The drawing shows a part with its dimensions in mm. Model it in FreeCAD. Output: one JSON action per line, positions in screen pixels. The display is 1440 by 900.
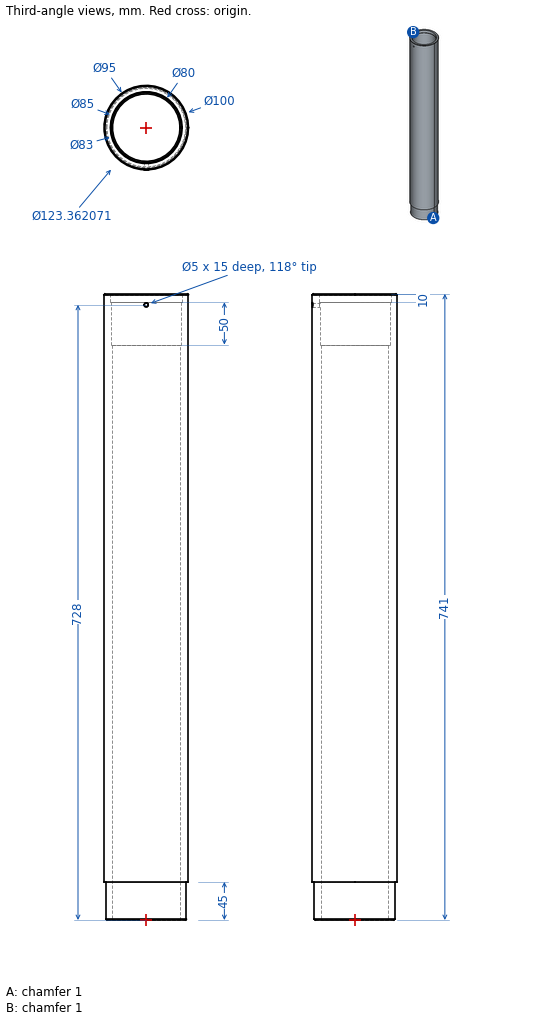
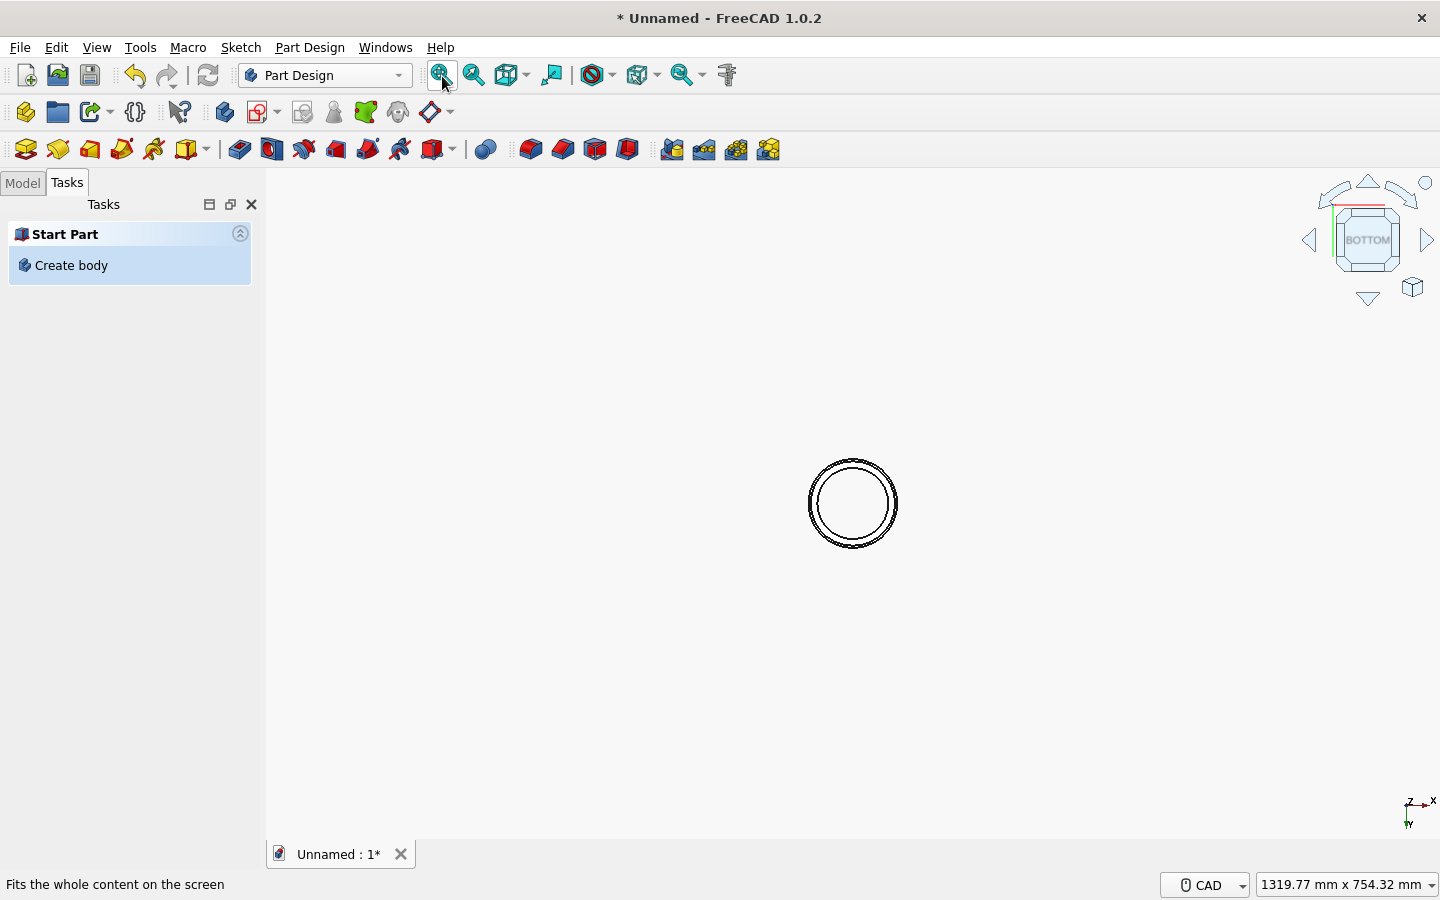
{"action": "left_click", "coordinate": [811, 502]}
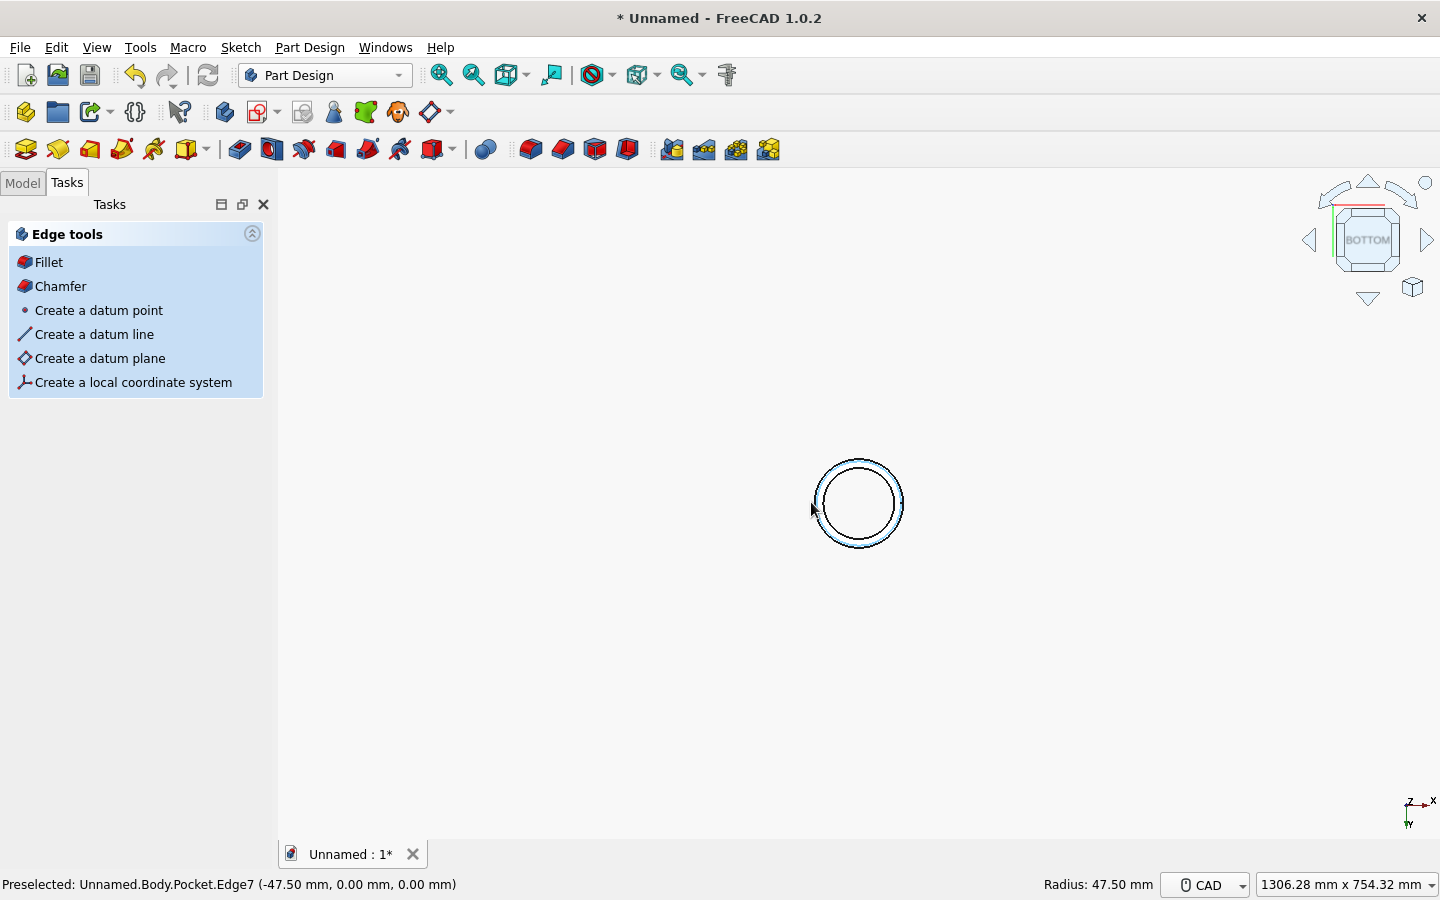
{"action": "left_click", "coordinate": [564, 150]}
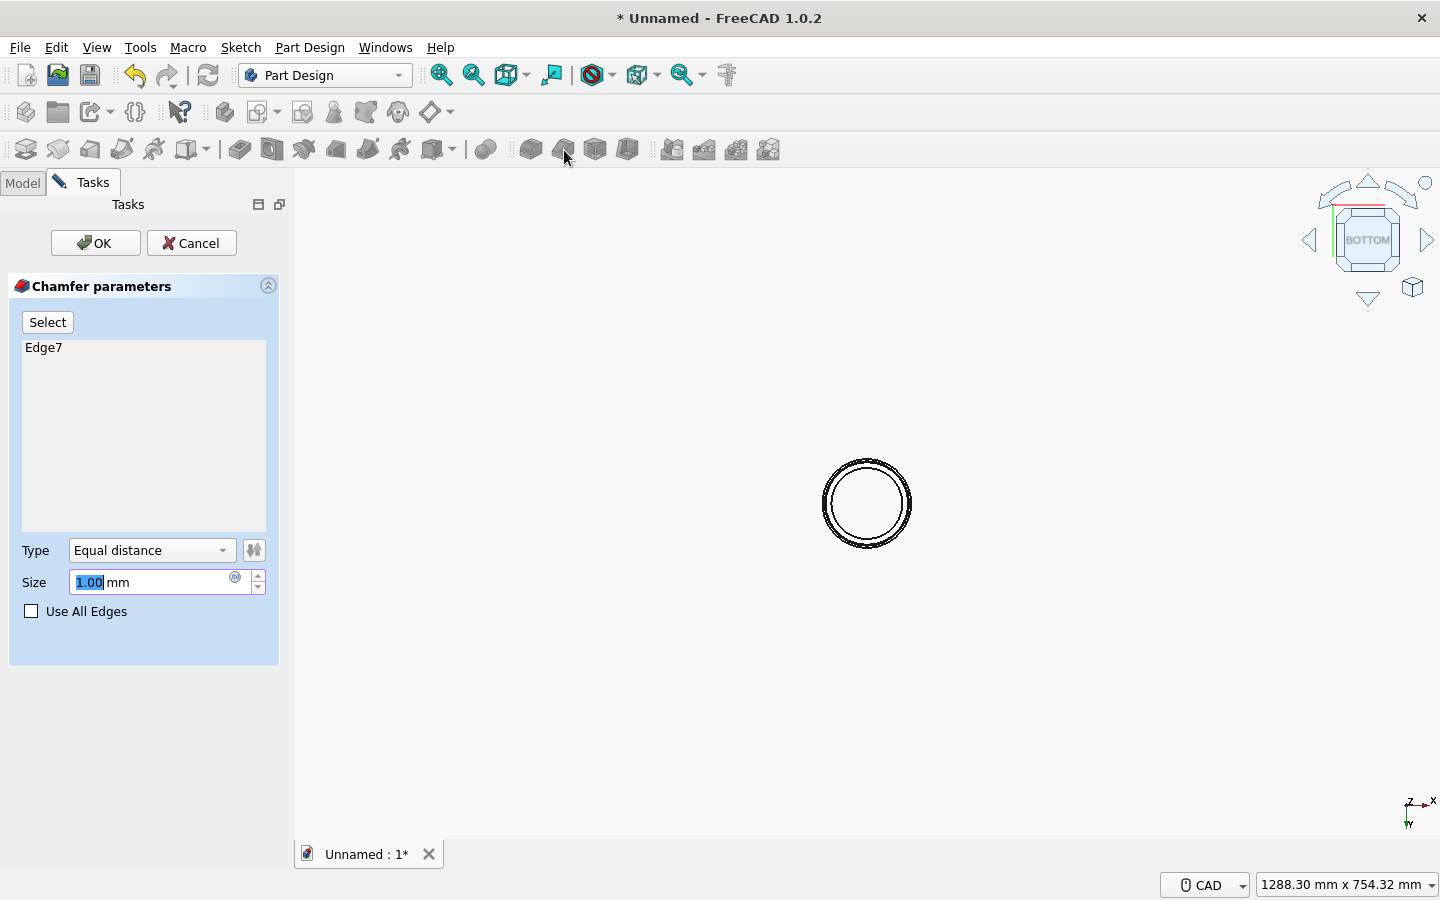
{"action": "type", "text": "1"}
{"action": "key", "text": "Tab"}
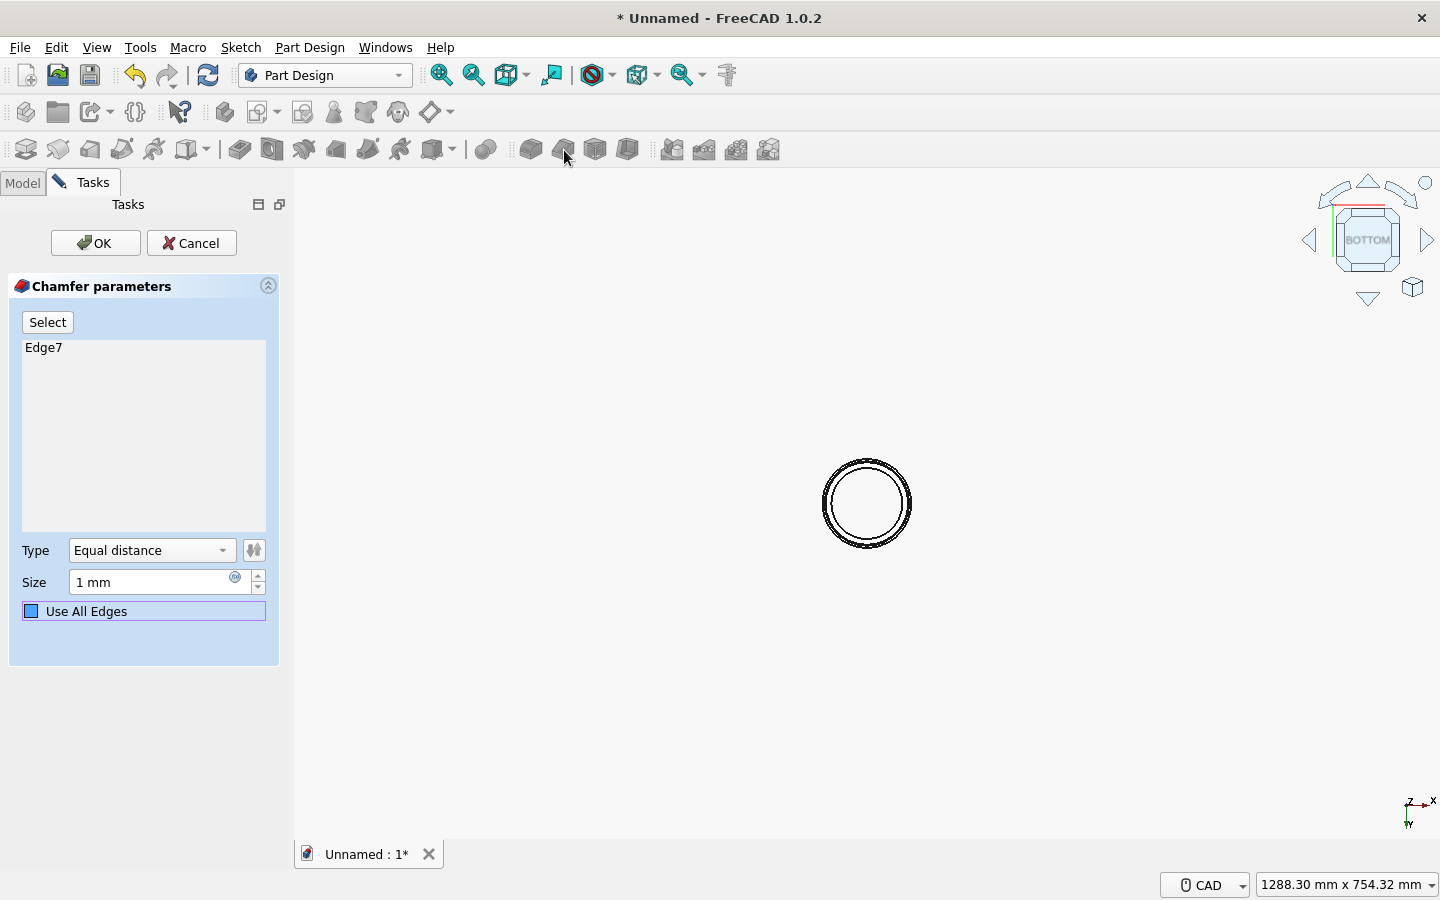
{"action": "left_click", "coordinate": [96, 243]}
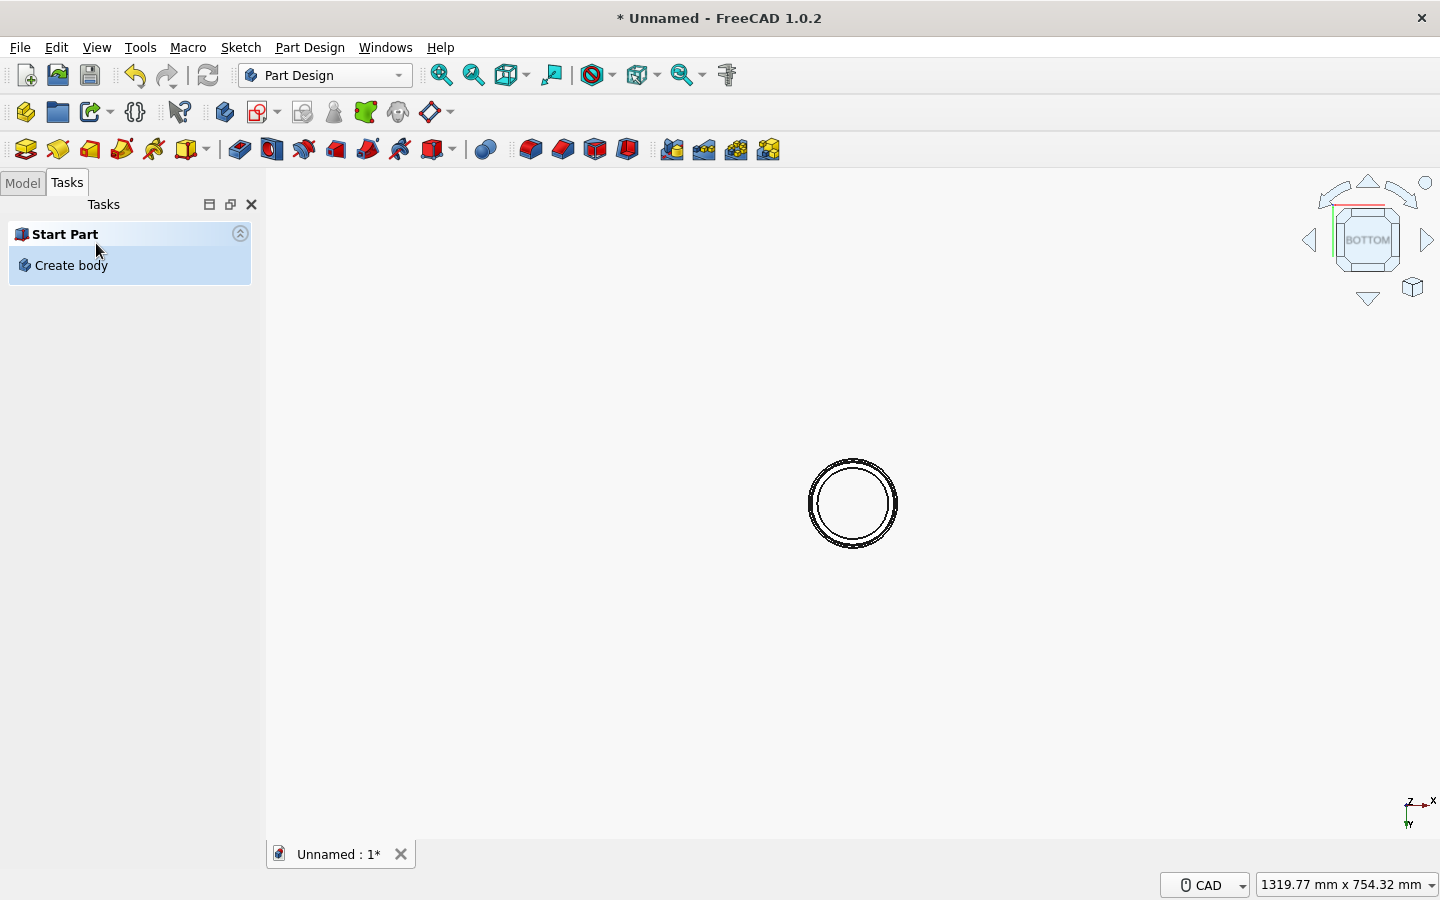
{"action": "left_click", "coordinate": [442, 76]}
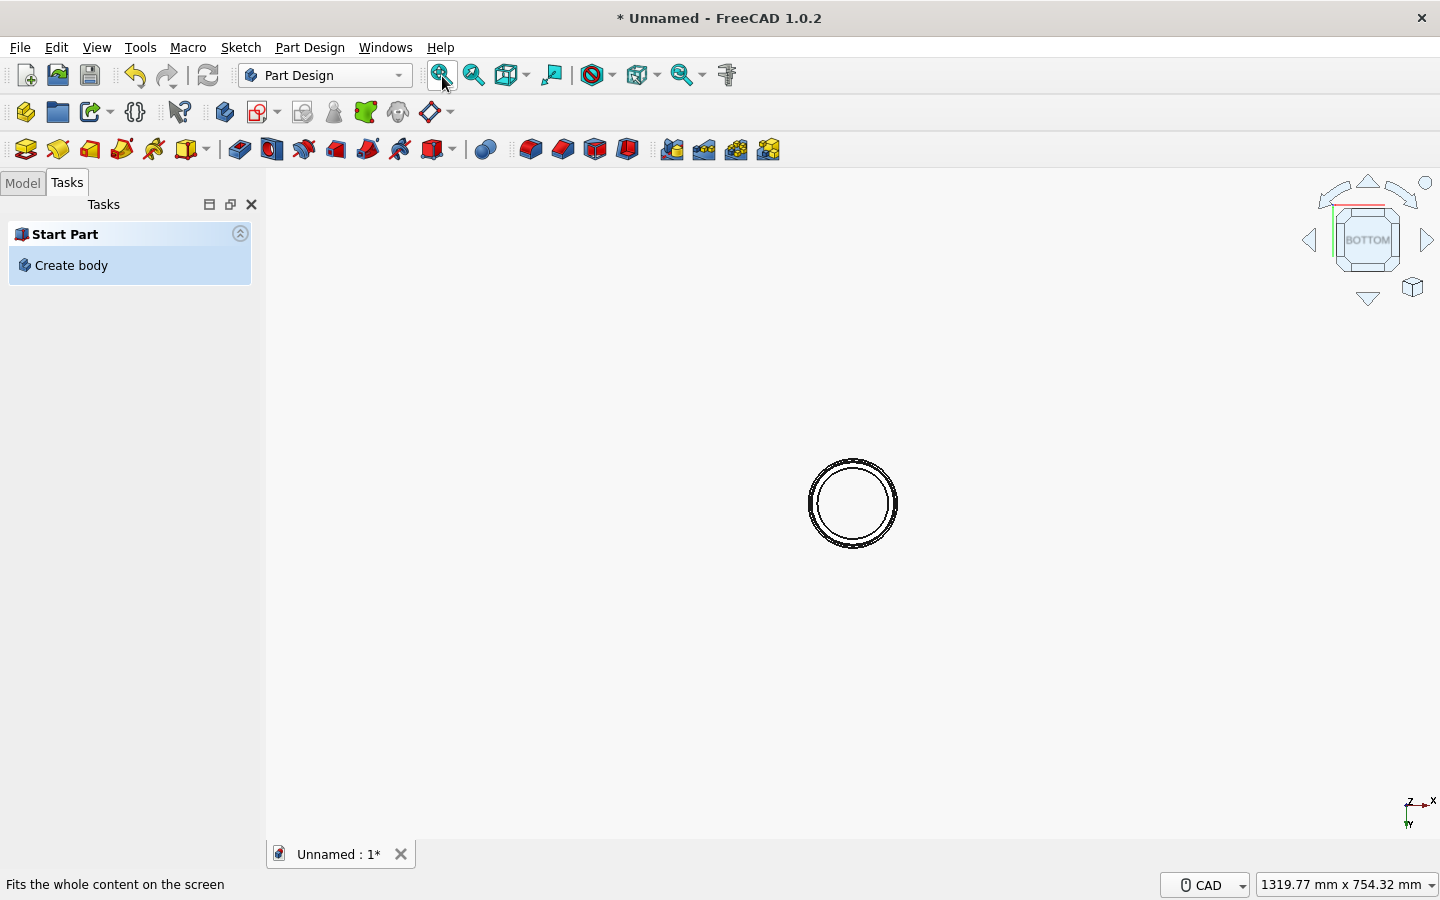
{"action": "key", "text": "0"}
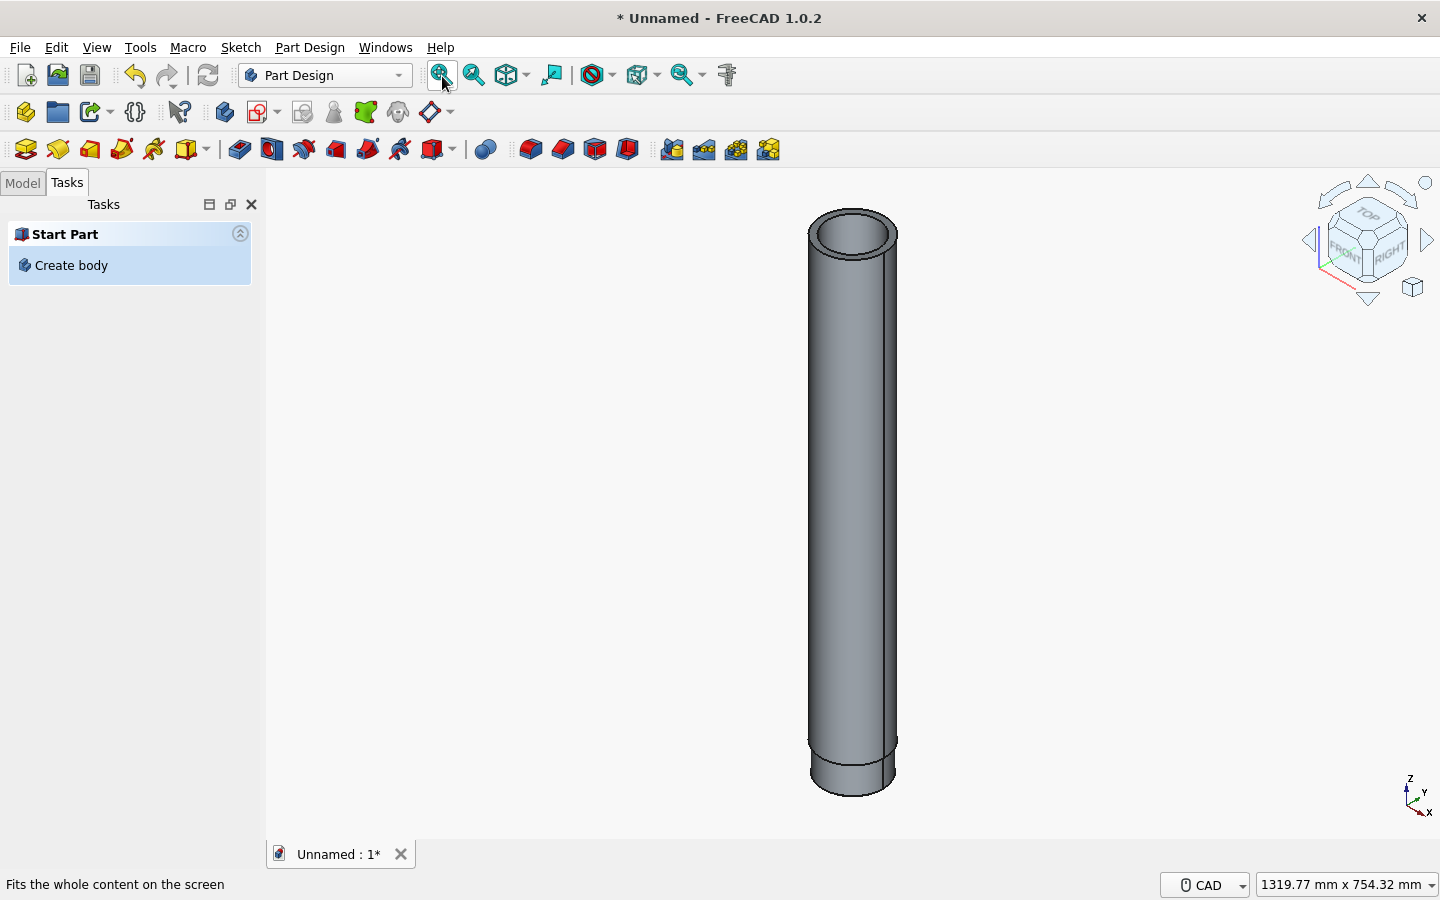
{"action": "left_click", "coordinate": [813, 245]}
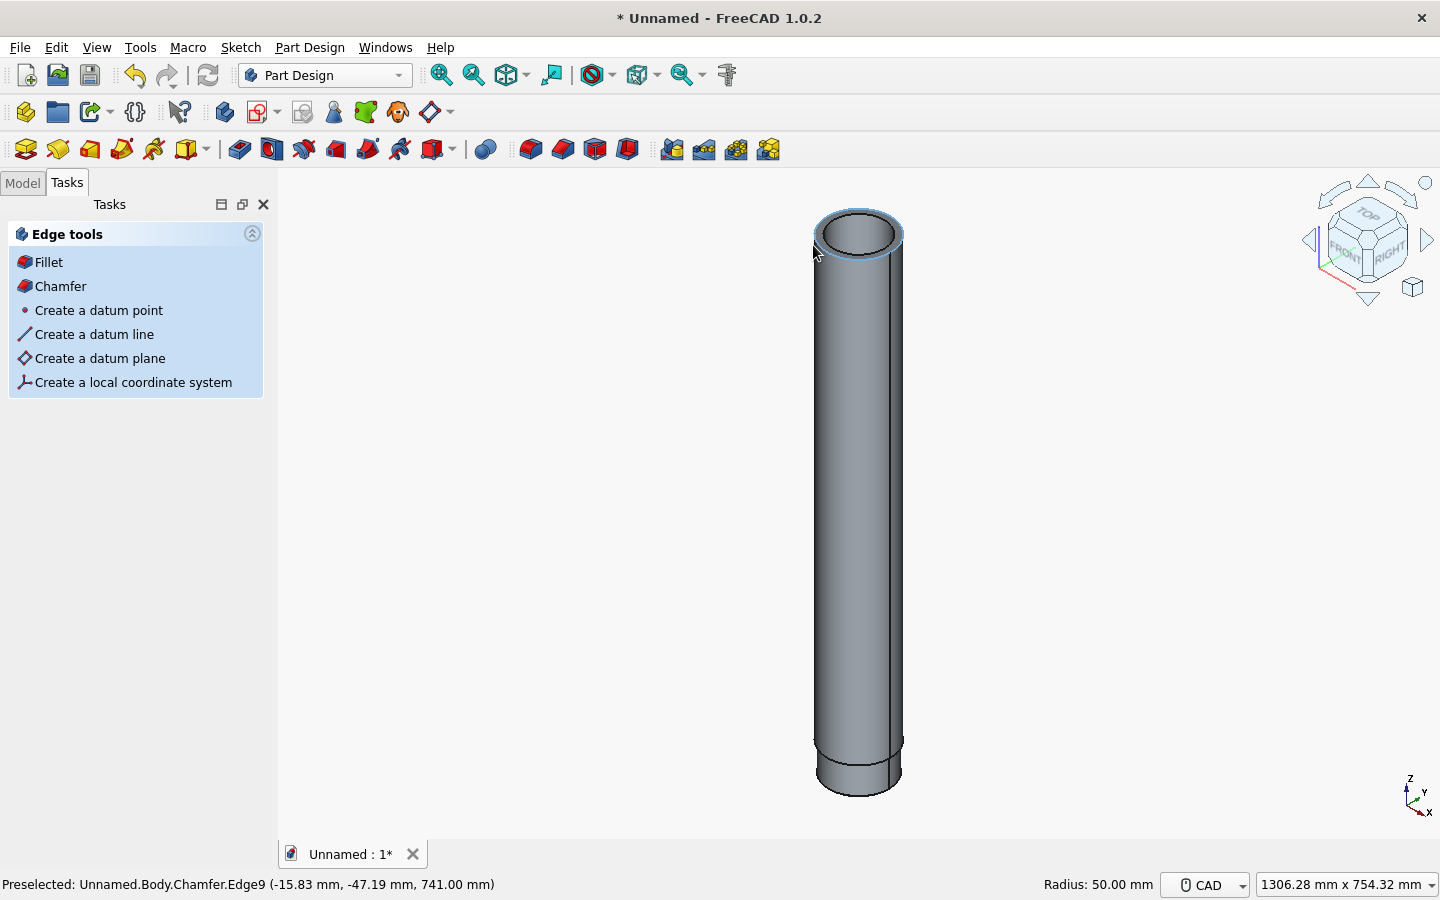
{"action": "left_click", "coordinate": [564, 150]}